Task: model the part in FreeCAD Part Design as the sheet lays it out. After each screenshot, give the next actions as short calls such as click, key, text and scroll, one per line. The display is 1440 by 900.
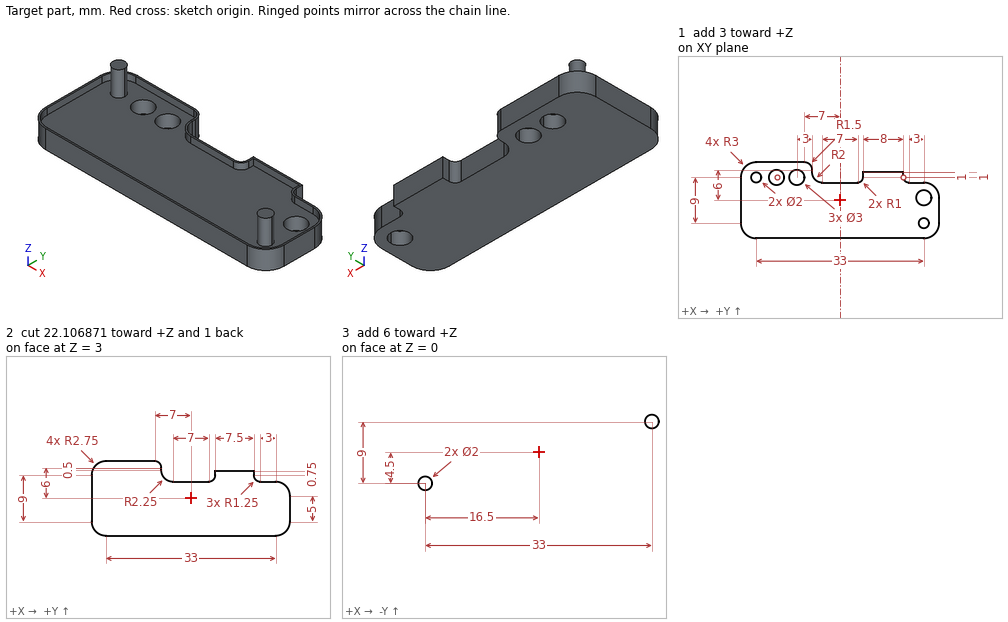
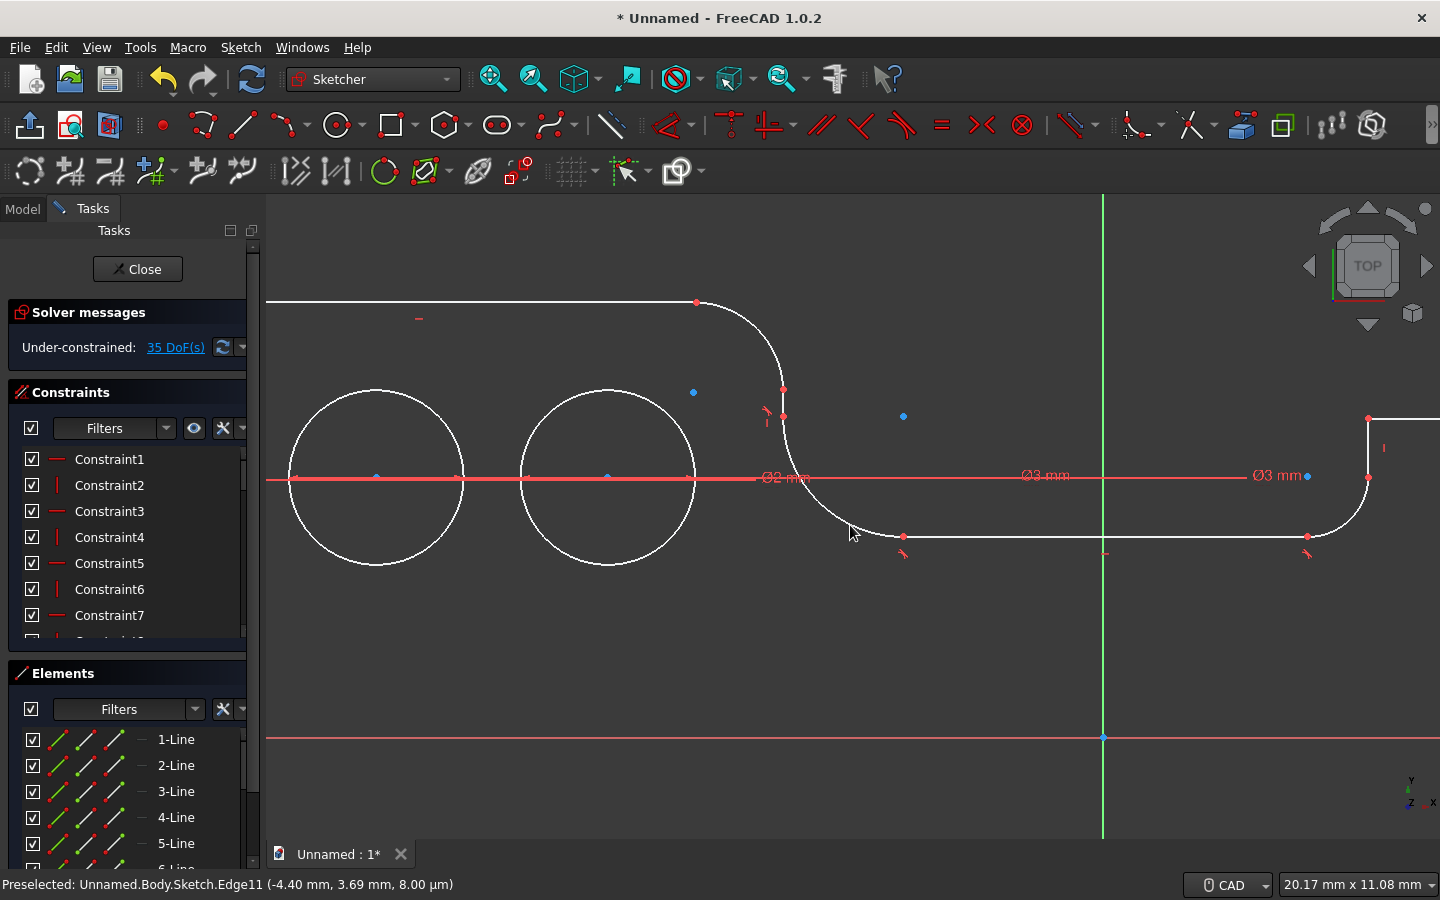
scroll(783, 406, up, 2)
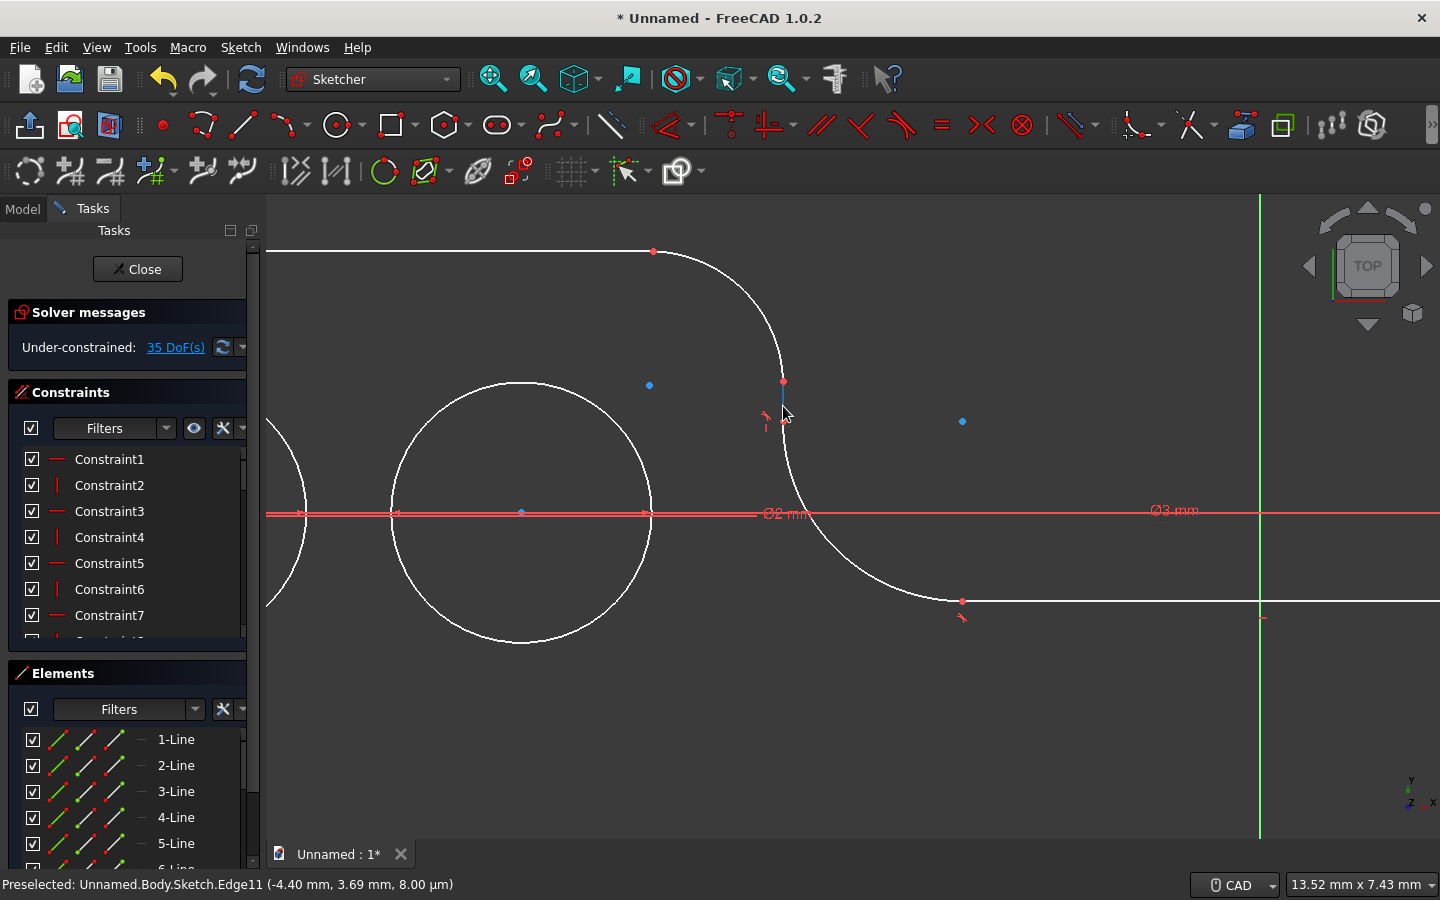
click(783, 406)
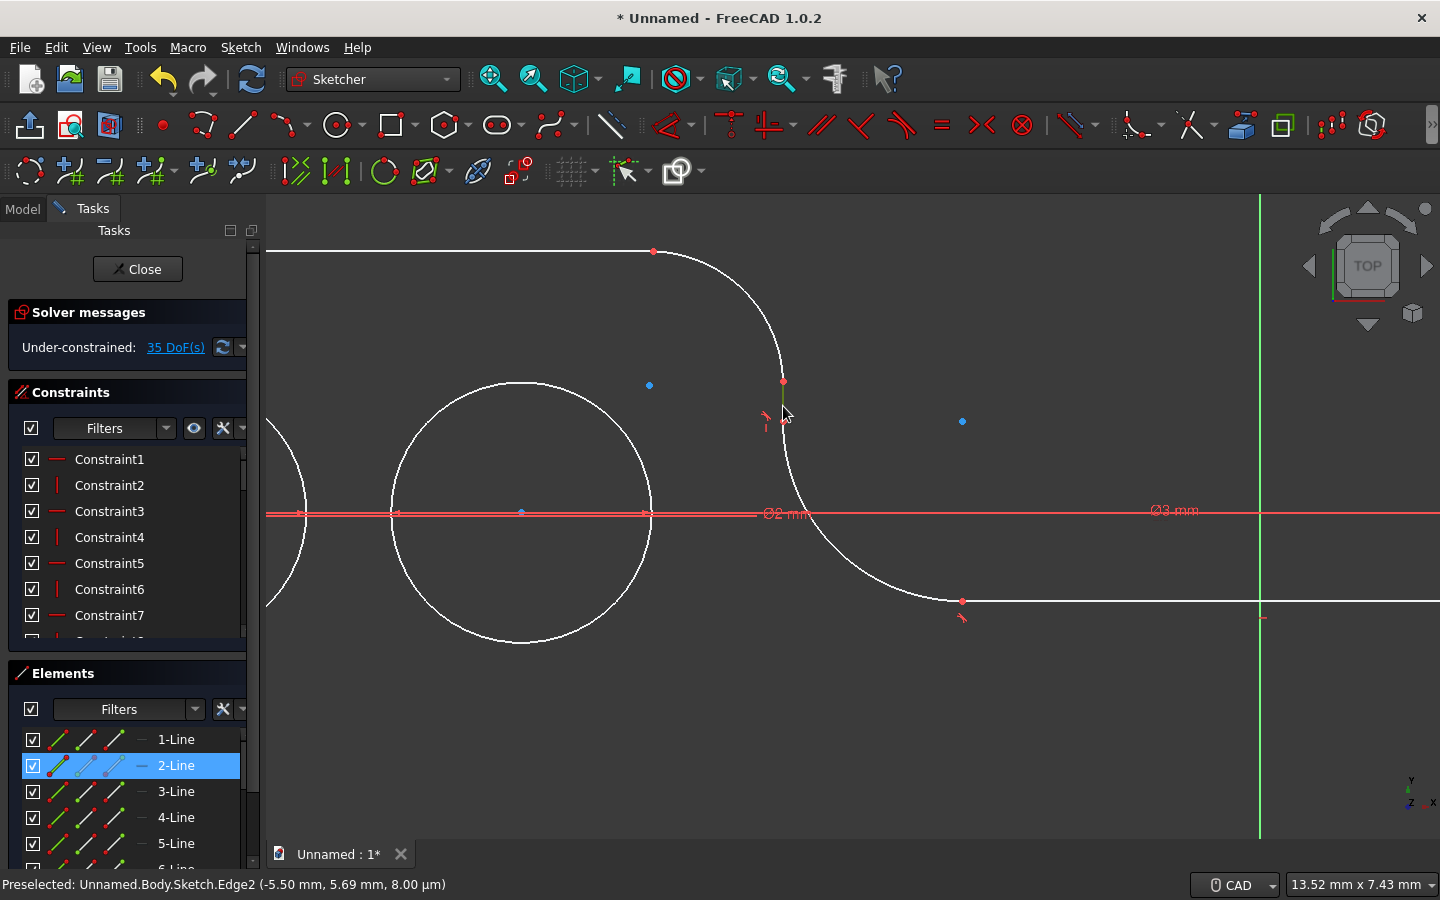
scroll(664, 419, down, 8)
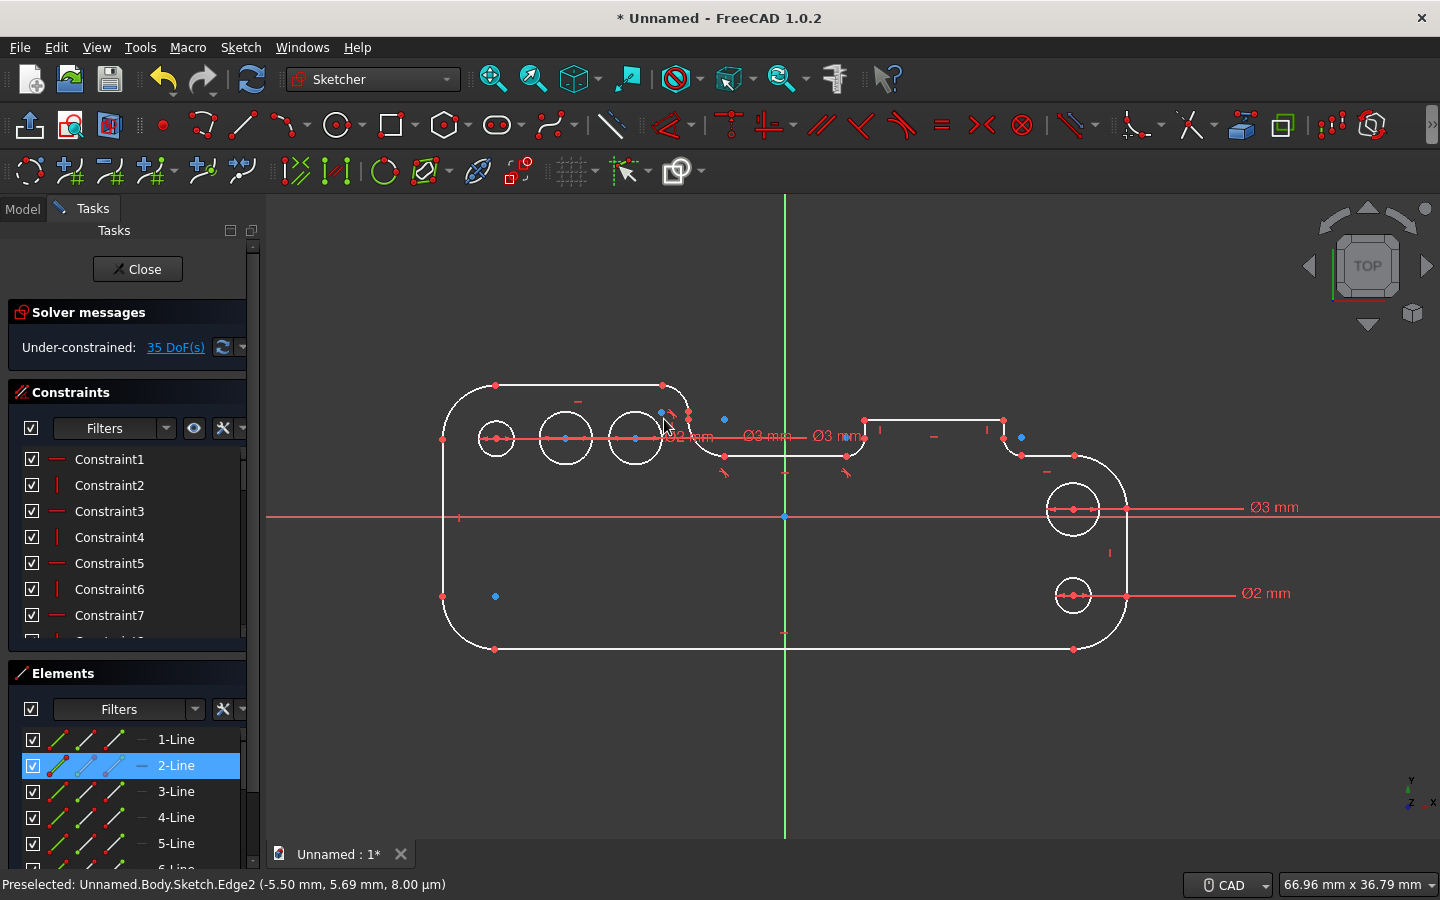
click(685, 400)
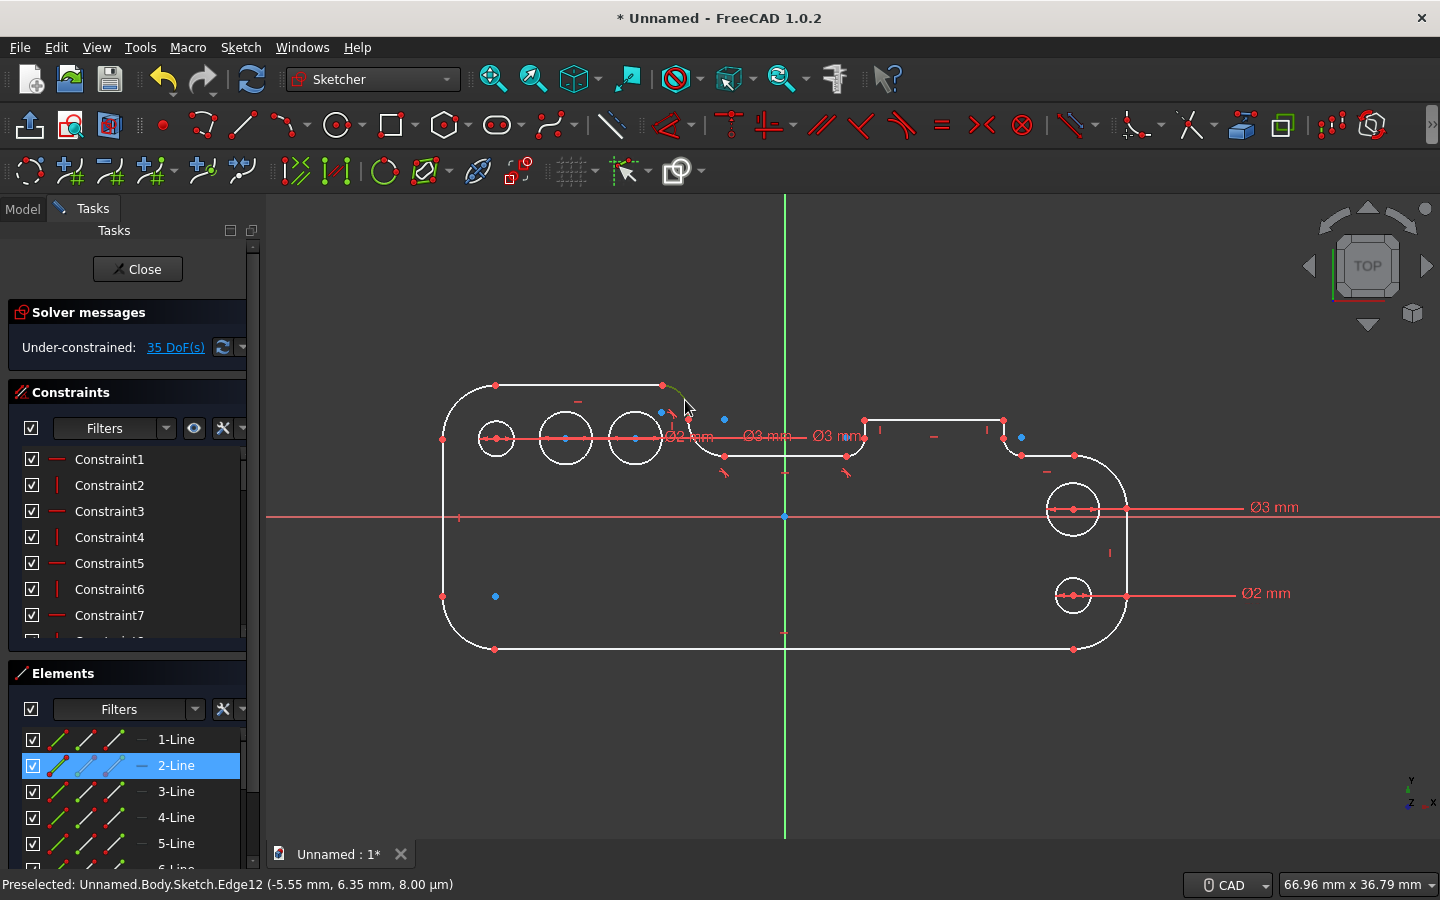
click(902, 126)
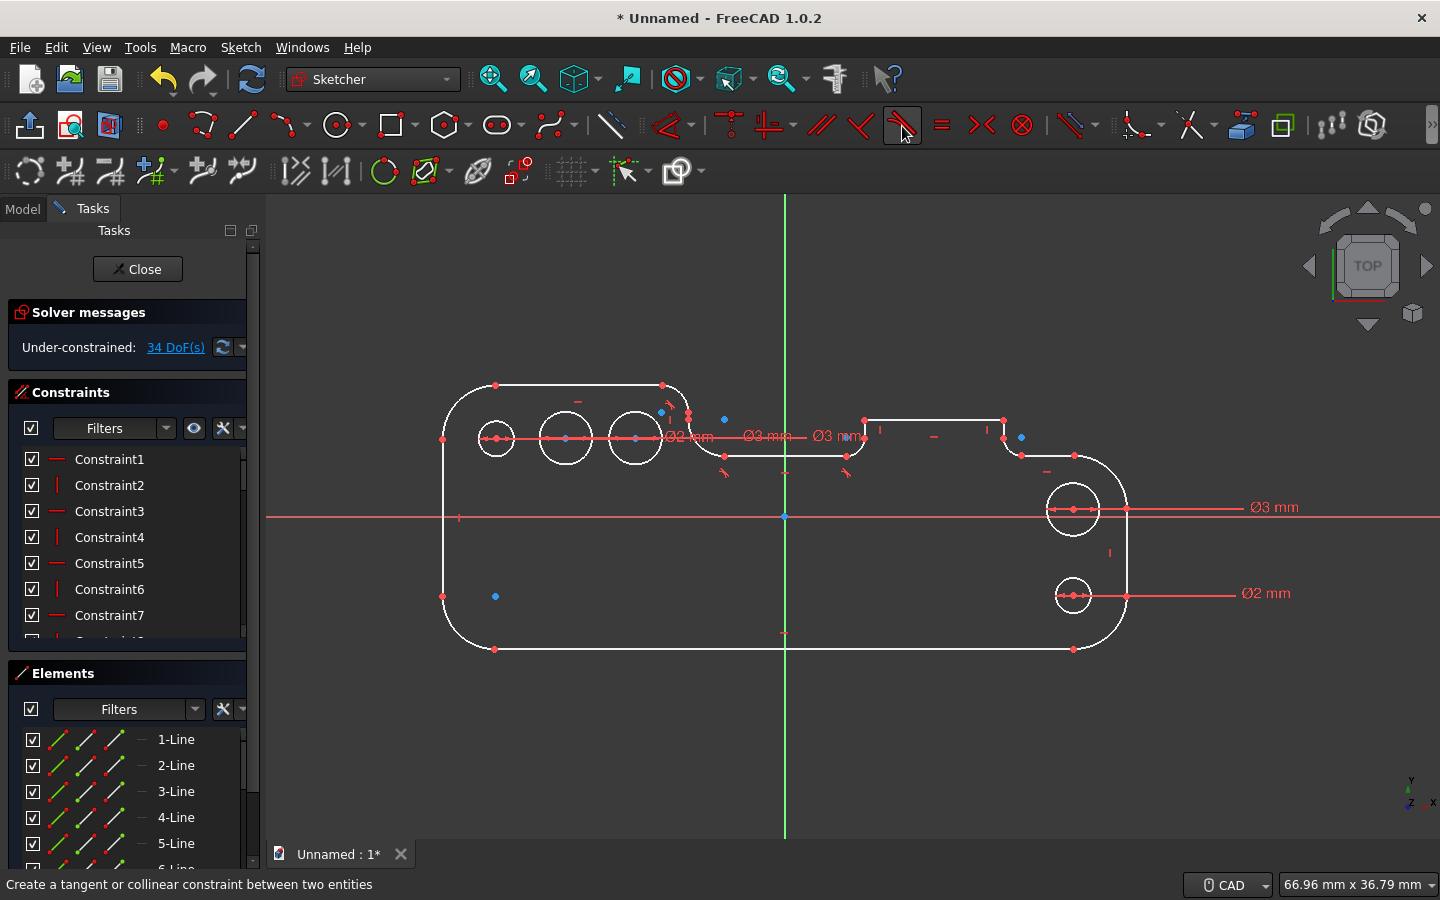
click(612, 385)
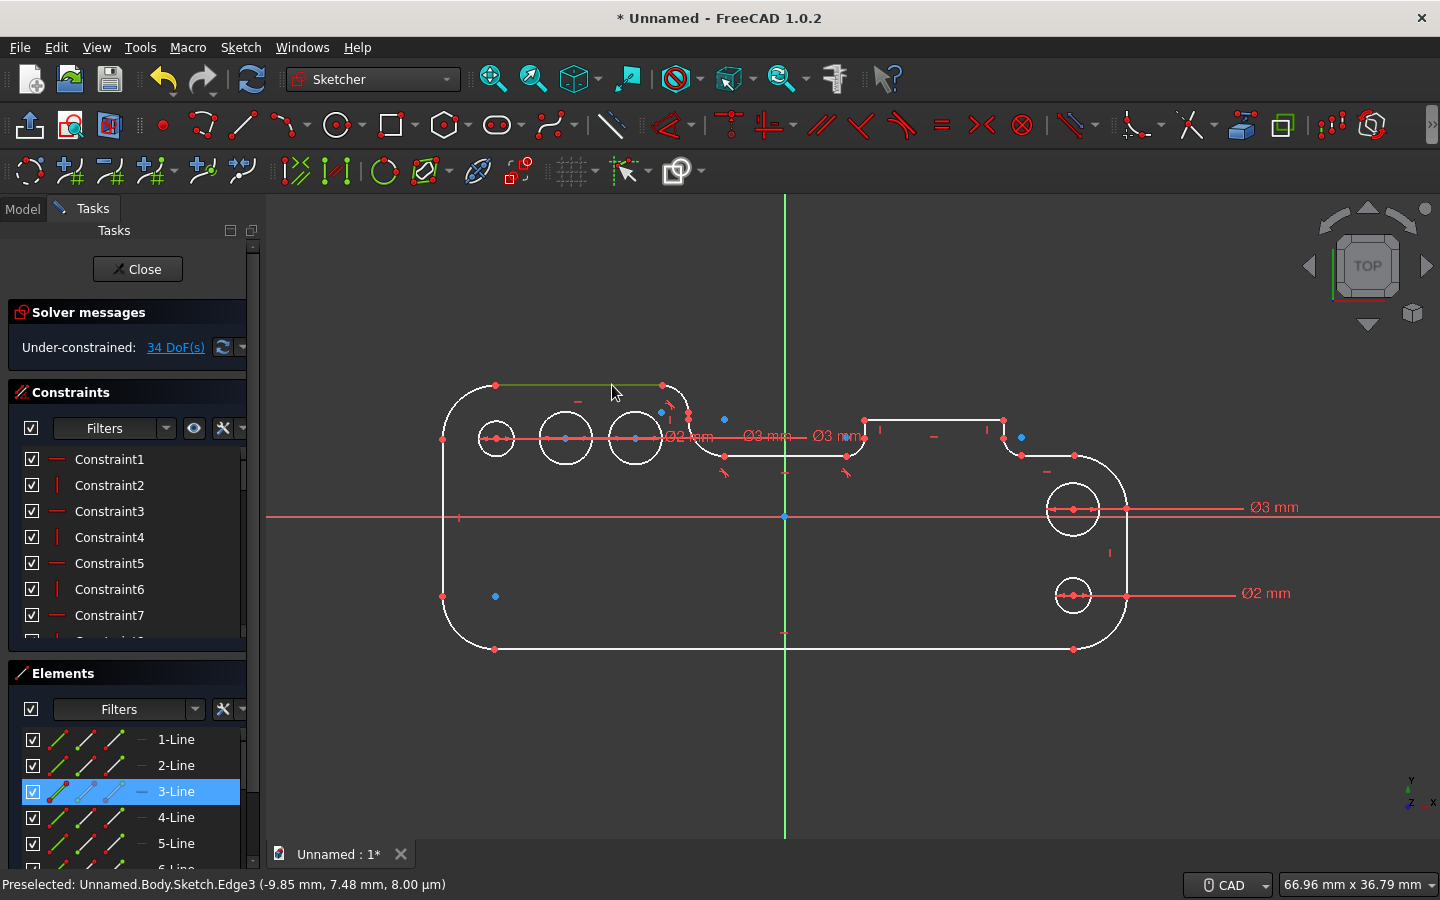
click(685, 400)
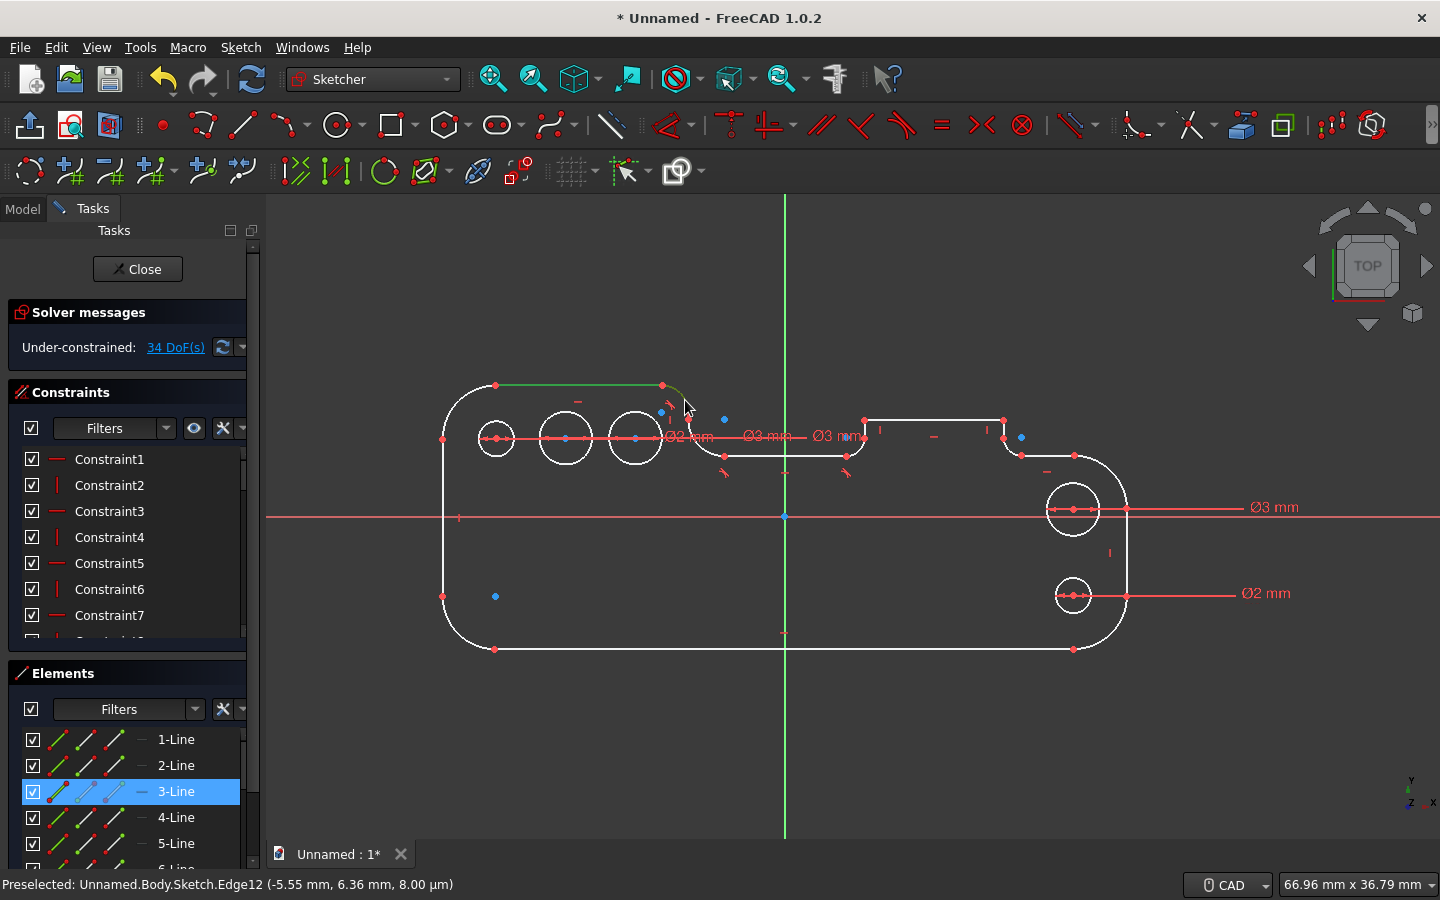
click(902, 126)